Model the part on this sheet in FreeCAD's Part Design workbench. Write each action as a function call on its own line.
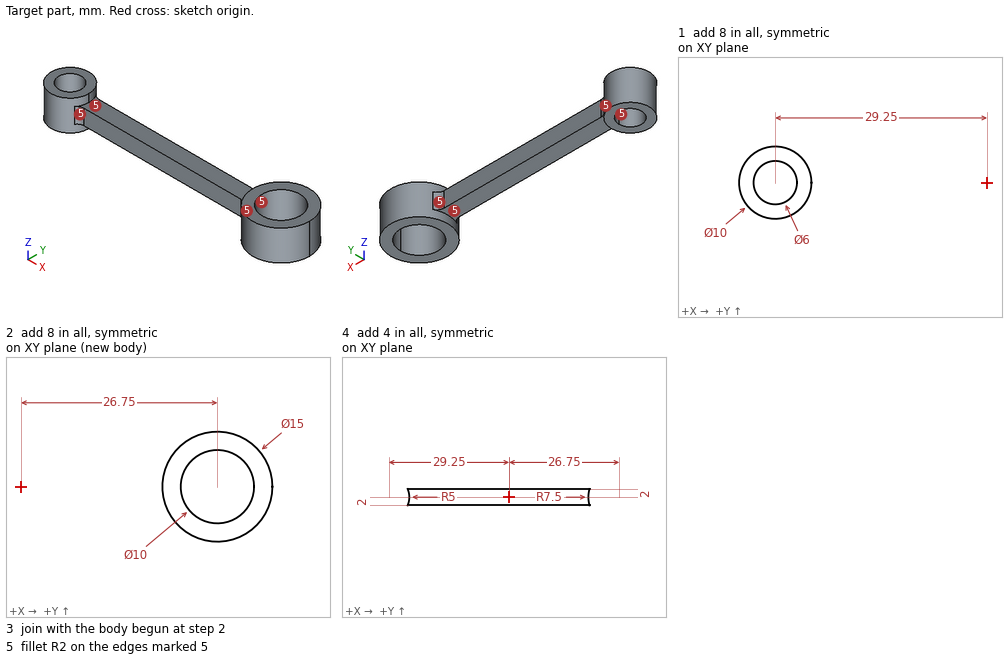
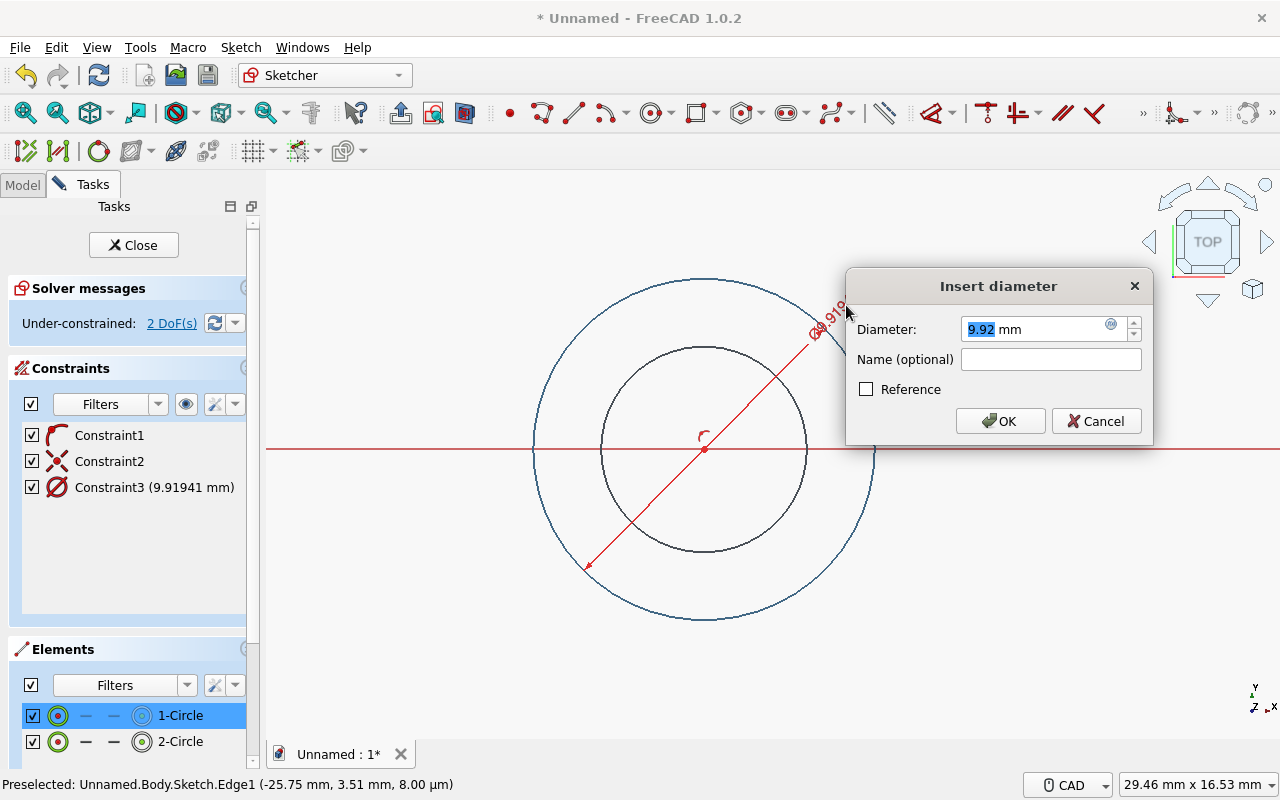
text(10)
key(Return)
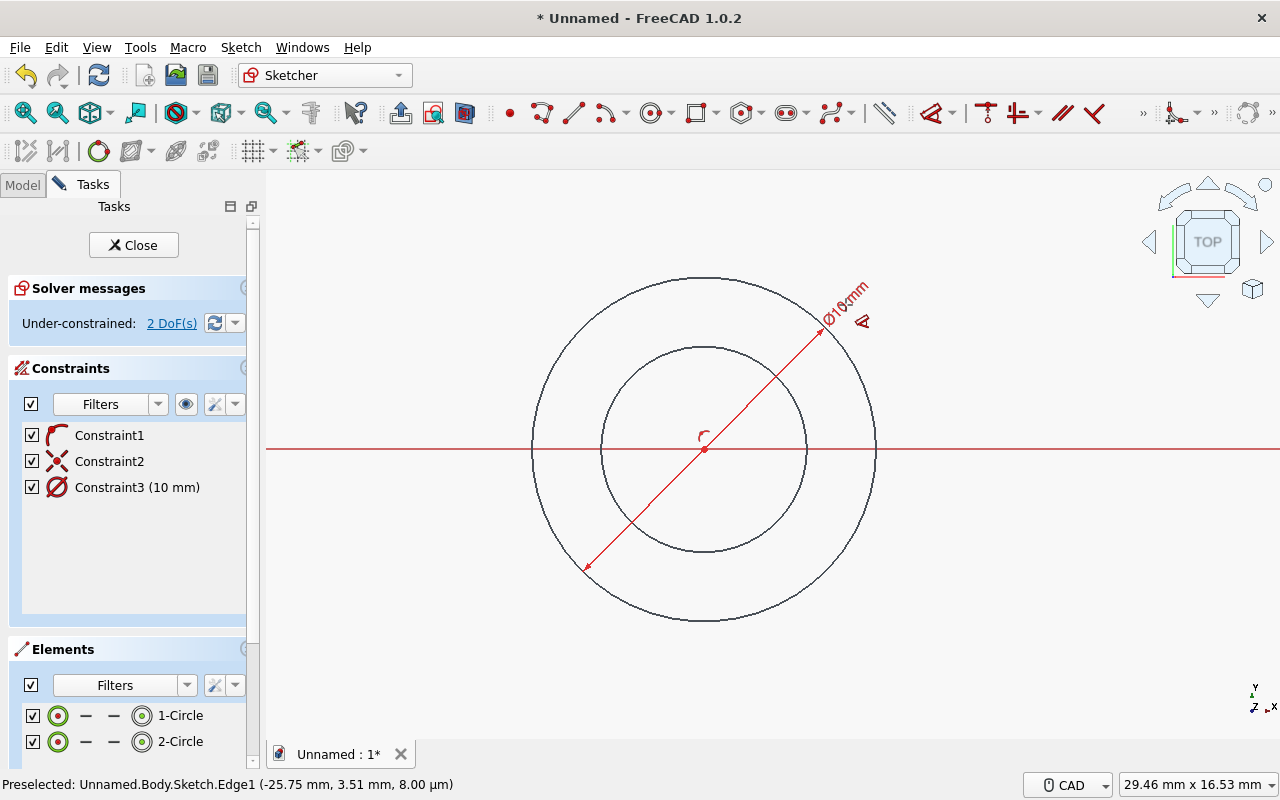
click(776, 376)
click(798, 353)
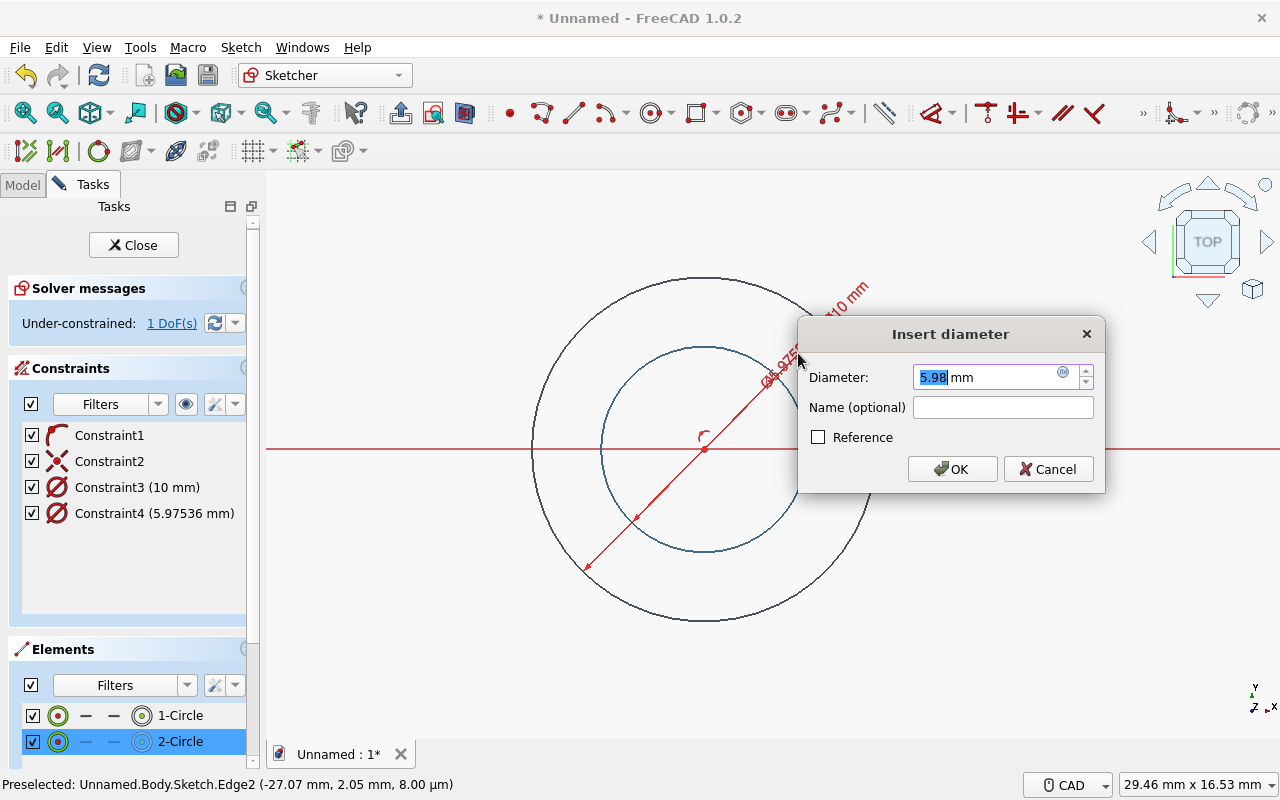
text(6)
key(Return)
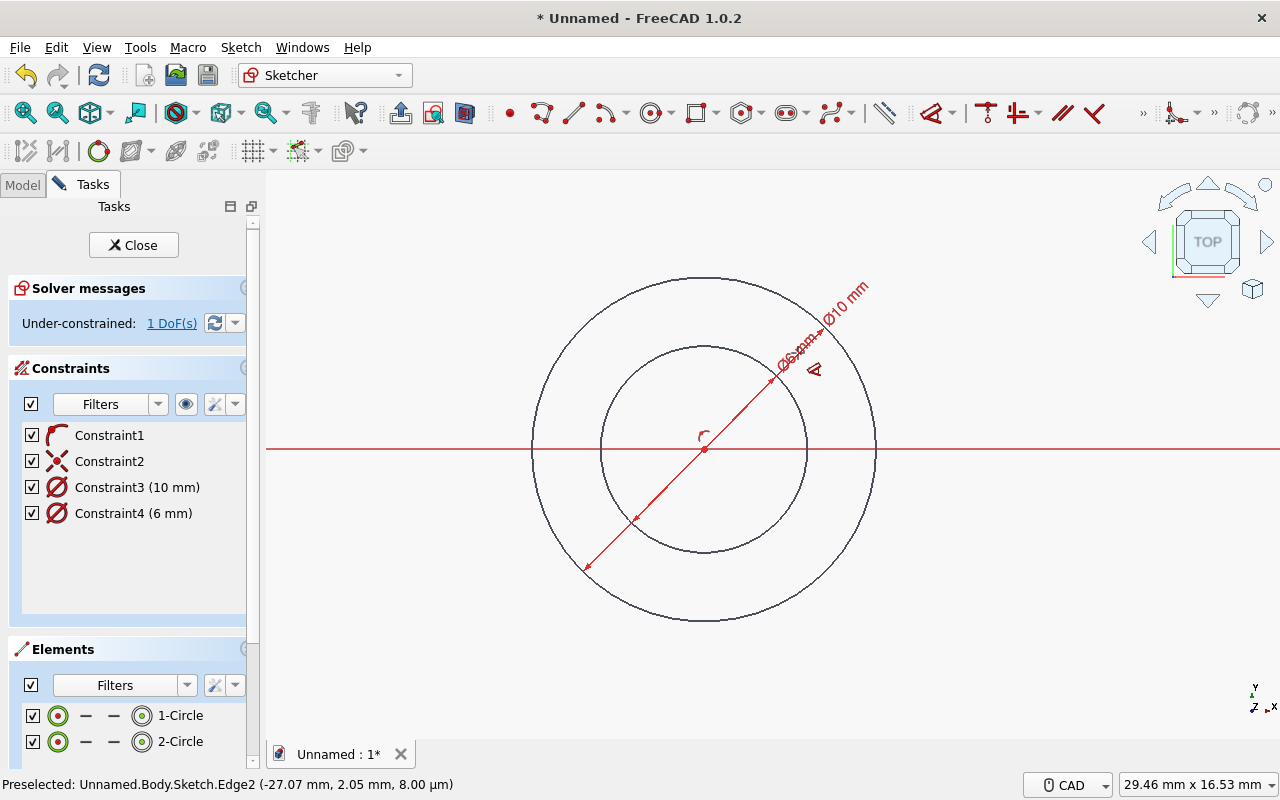
click(704, 449)
click(910, 483)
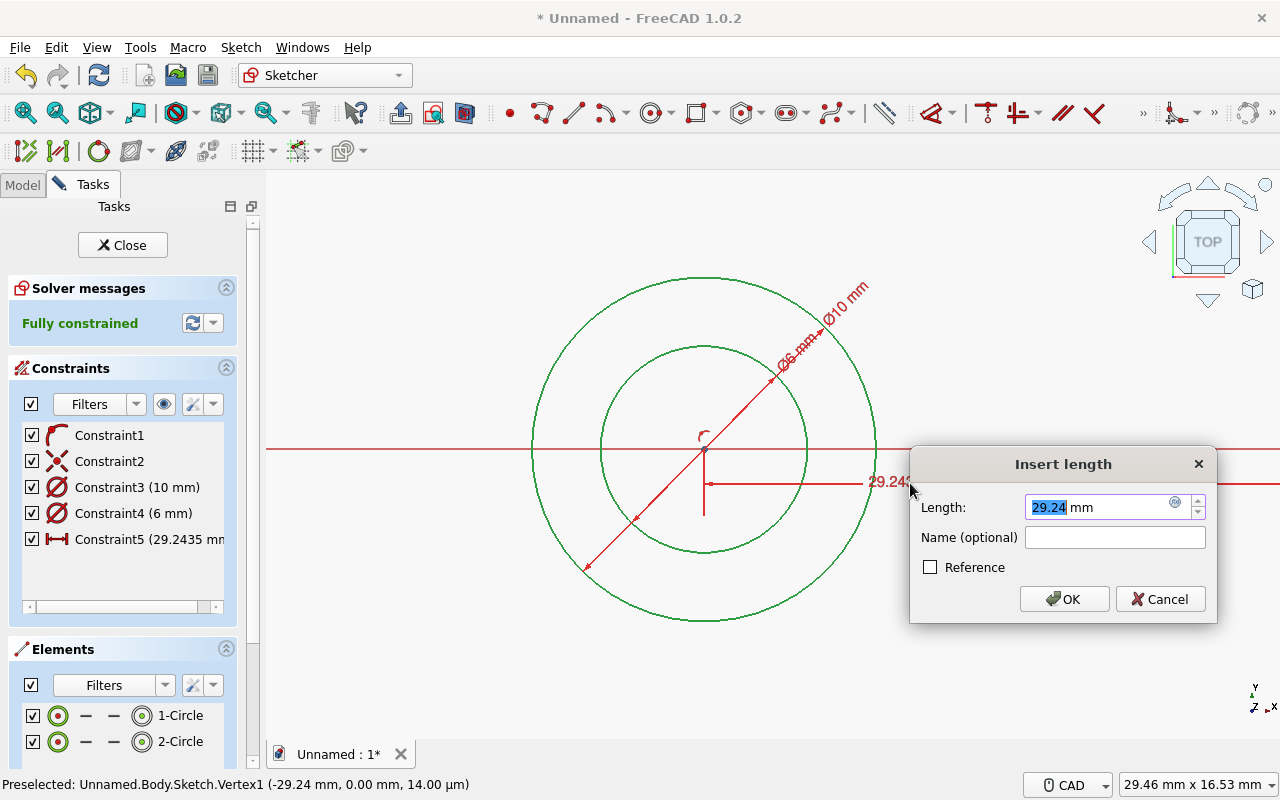
text(29.25)
key(Return)
key(Escape)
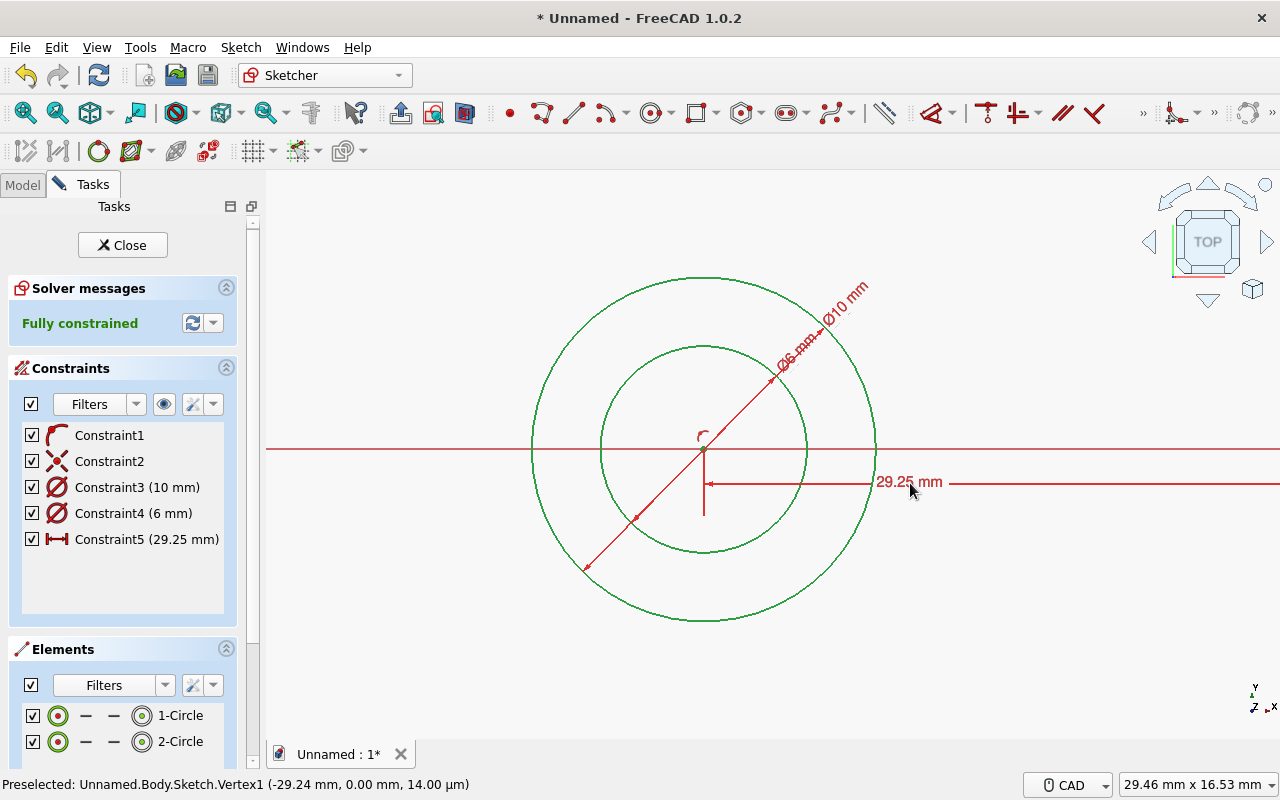
click(123, 245)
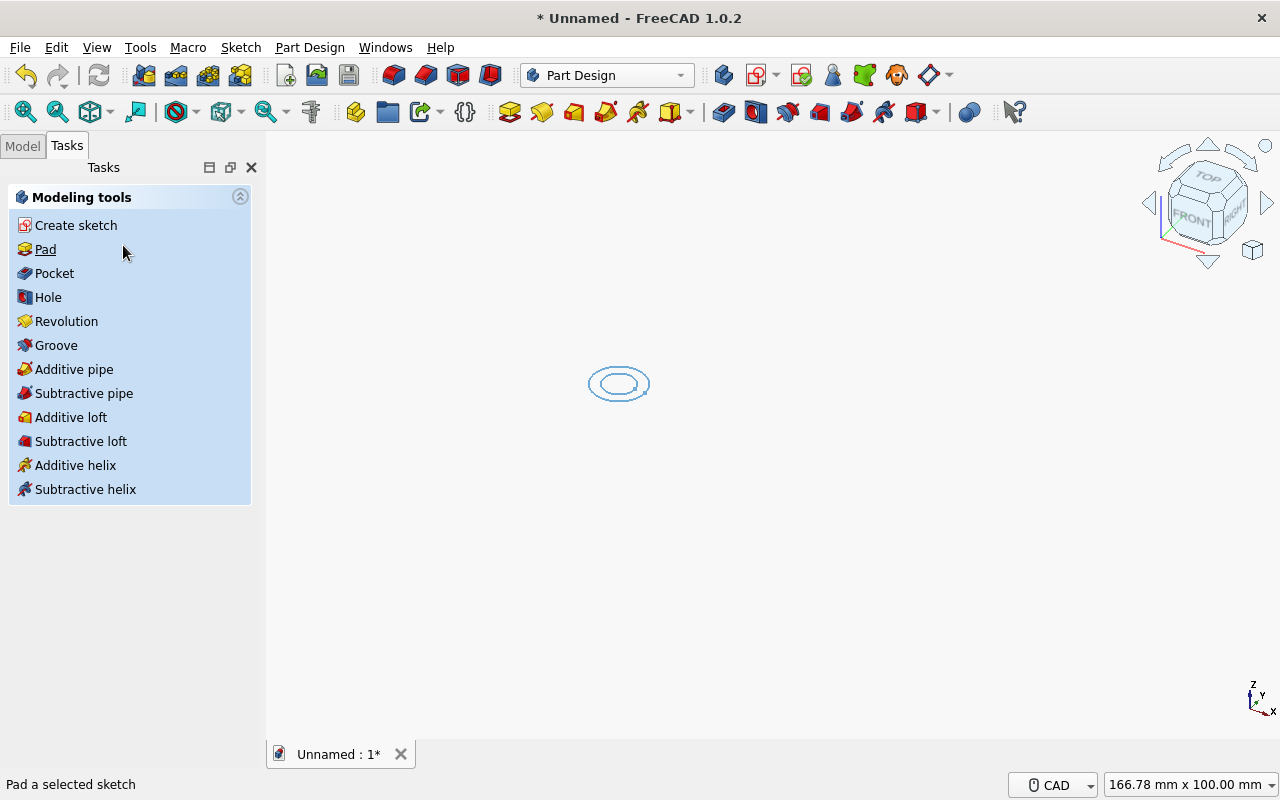
click(510, 112)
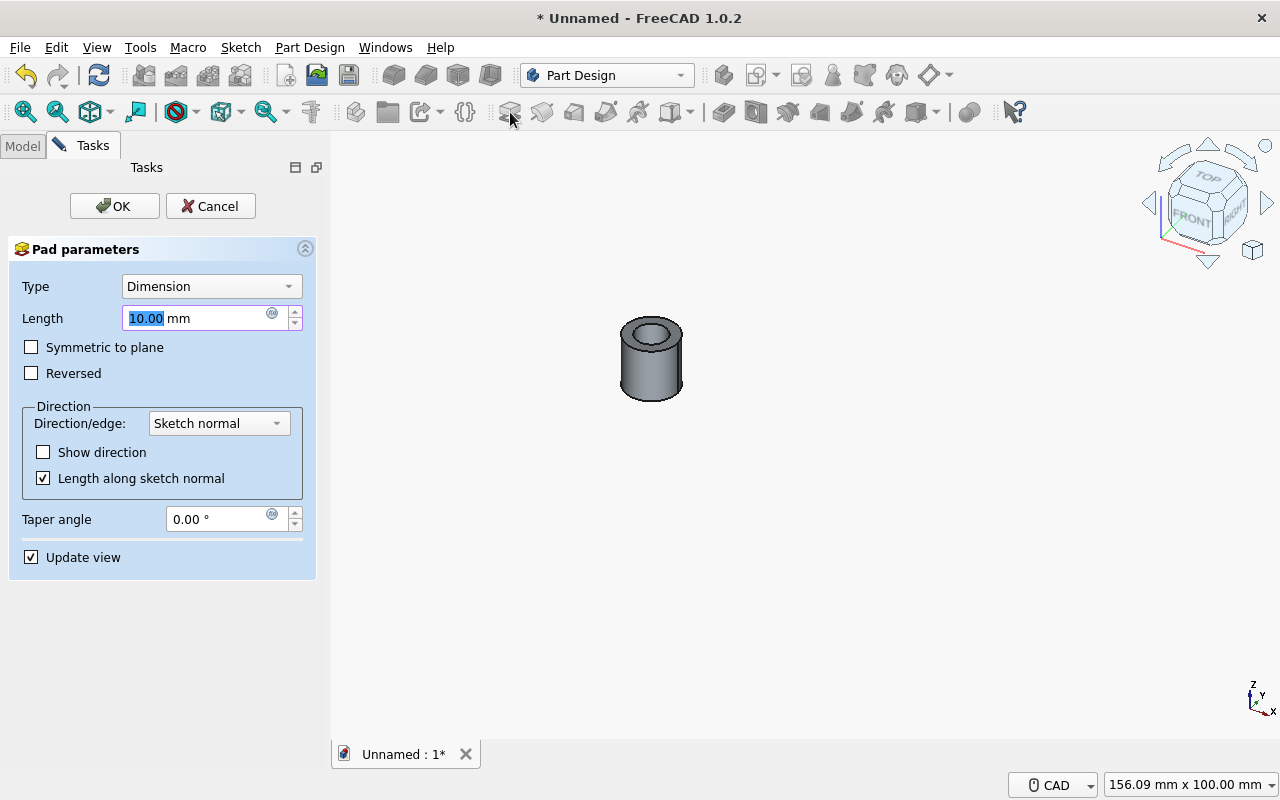
text(8)
key(Tab)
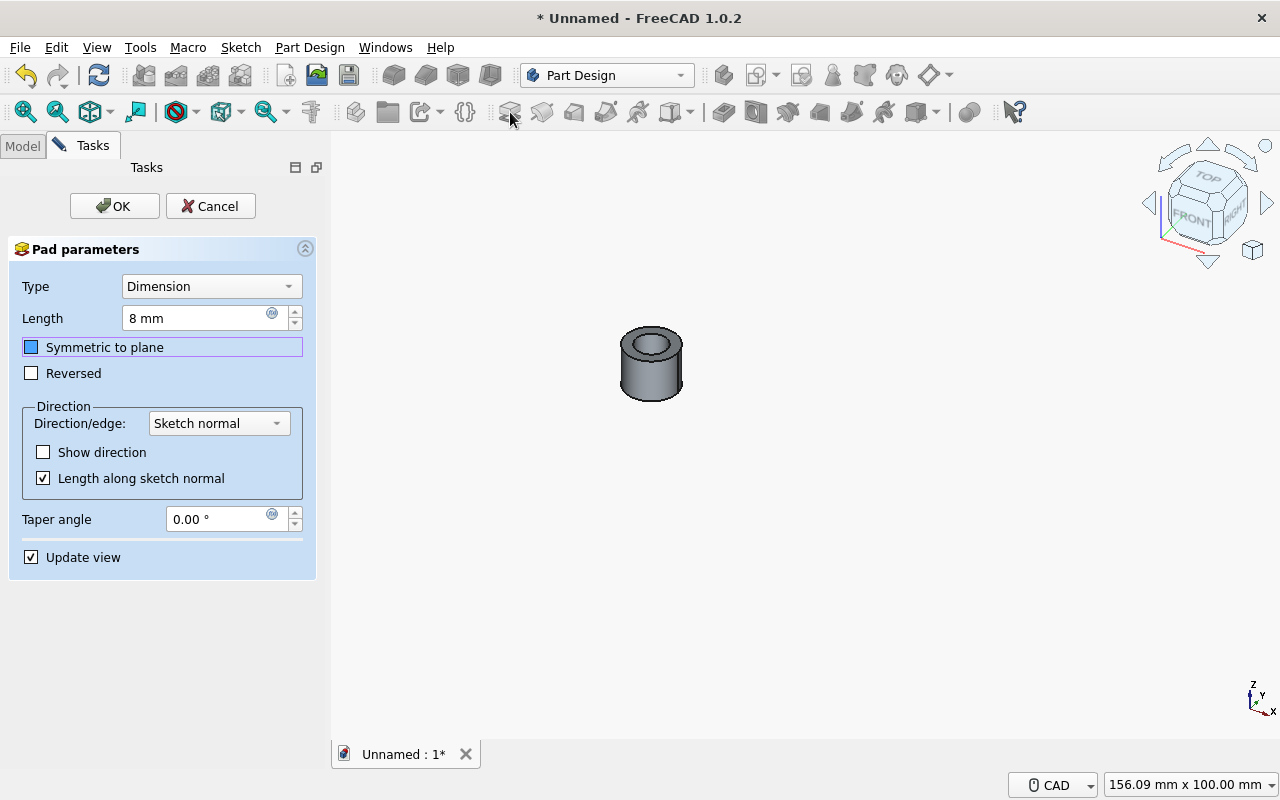
click(30, 347)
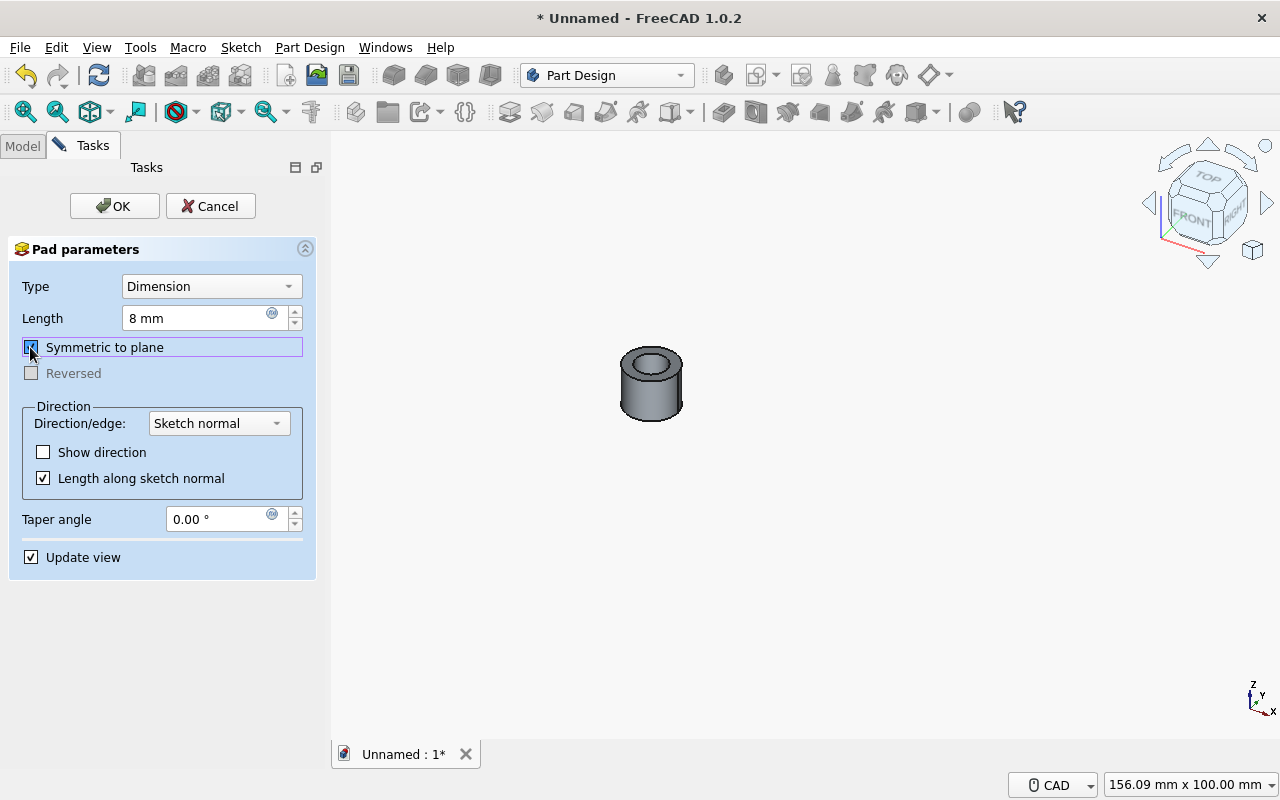
click(115, 206)